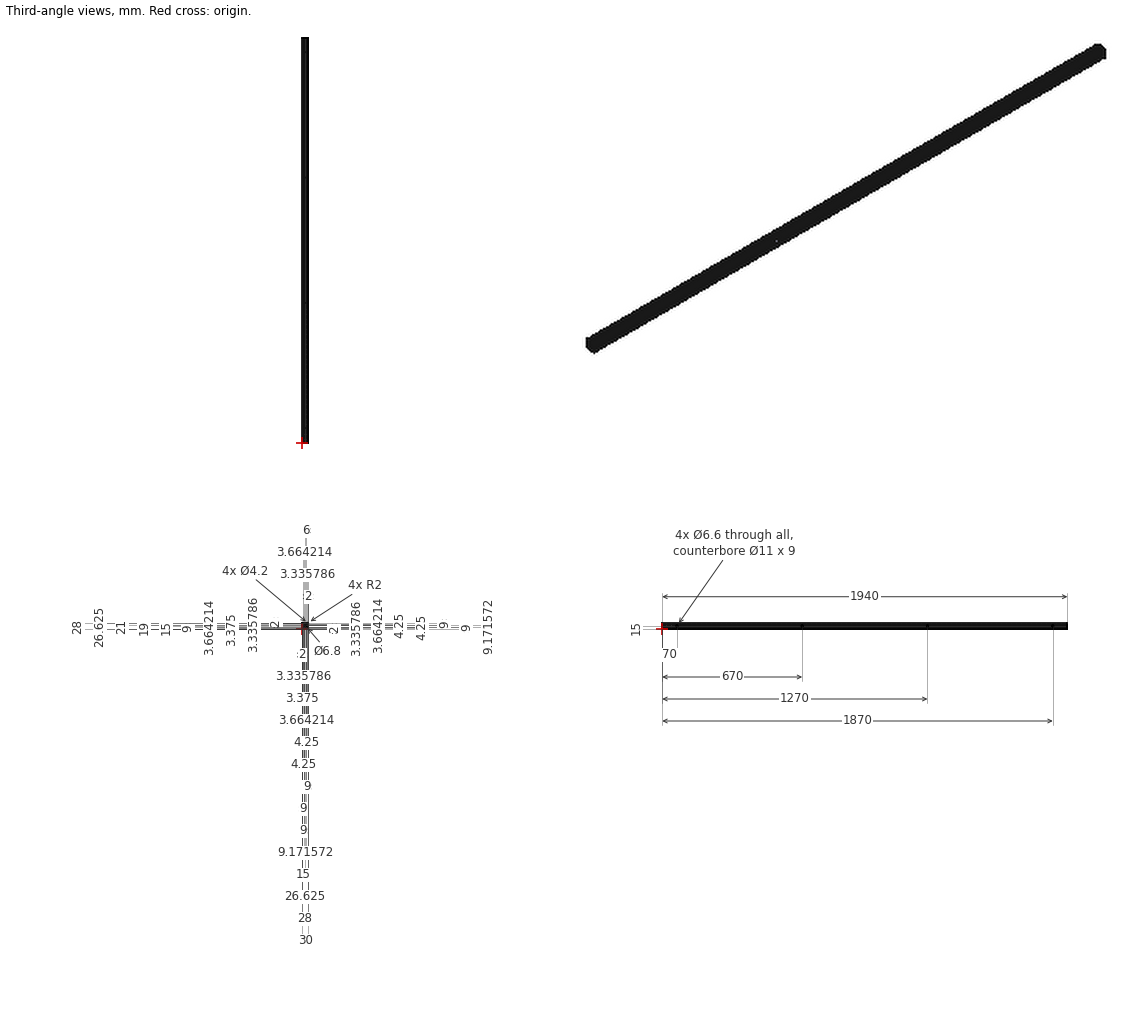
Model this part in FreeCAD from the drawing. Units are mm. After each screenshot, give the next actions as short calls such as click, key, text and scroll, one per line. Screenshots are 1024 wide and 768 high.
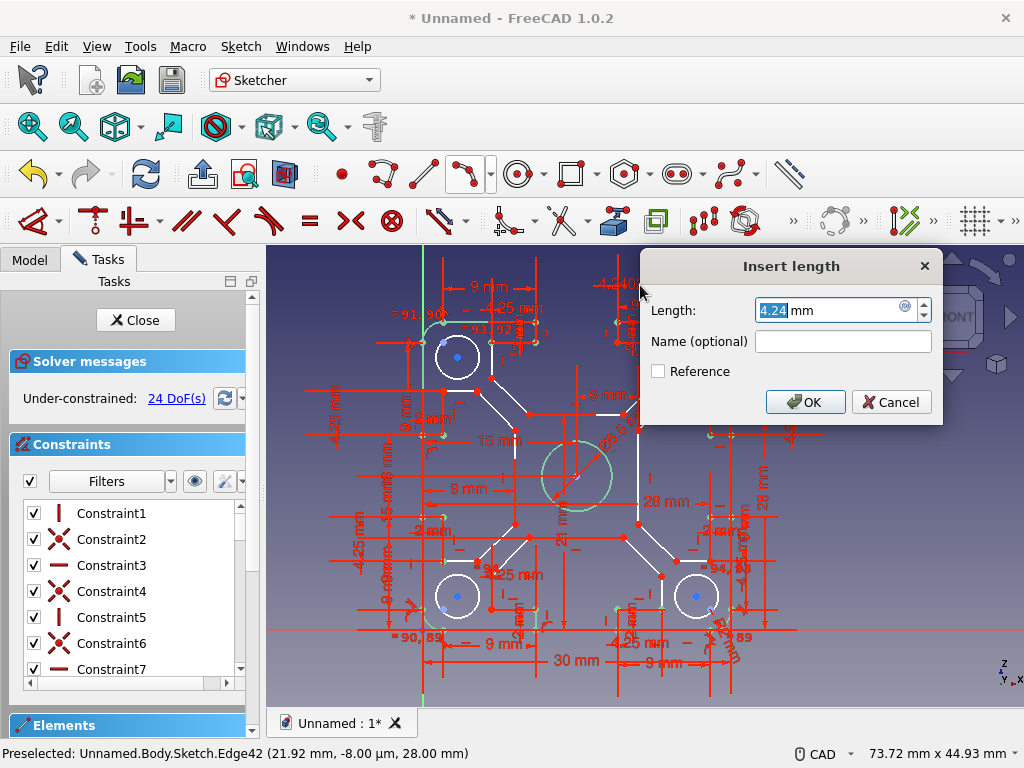
text(4.25)
key(Return)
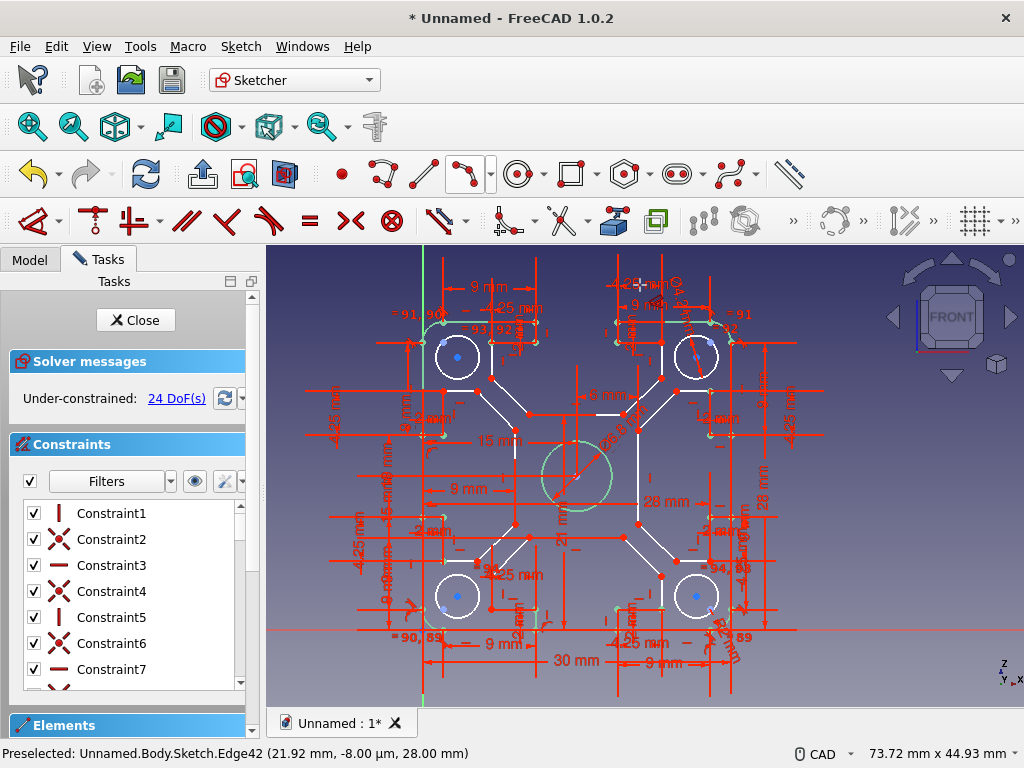
click(458, 357)
click(440, 664)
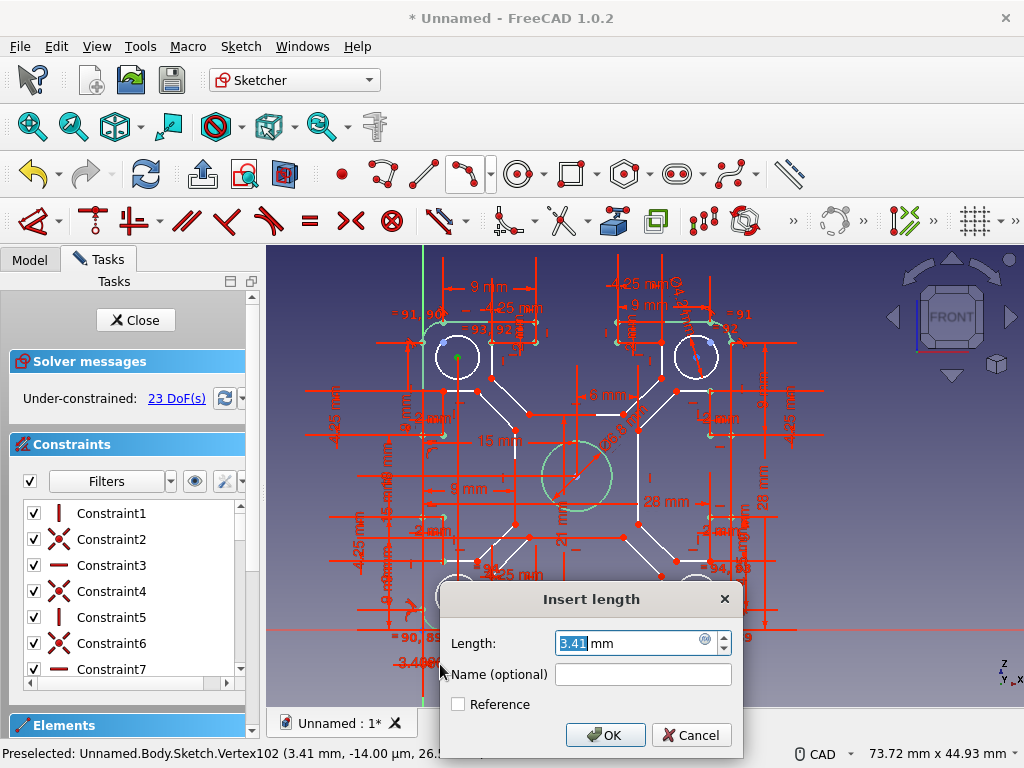
text(3.375)
key(Return)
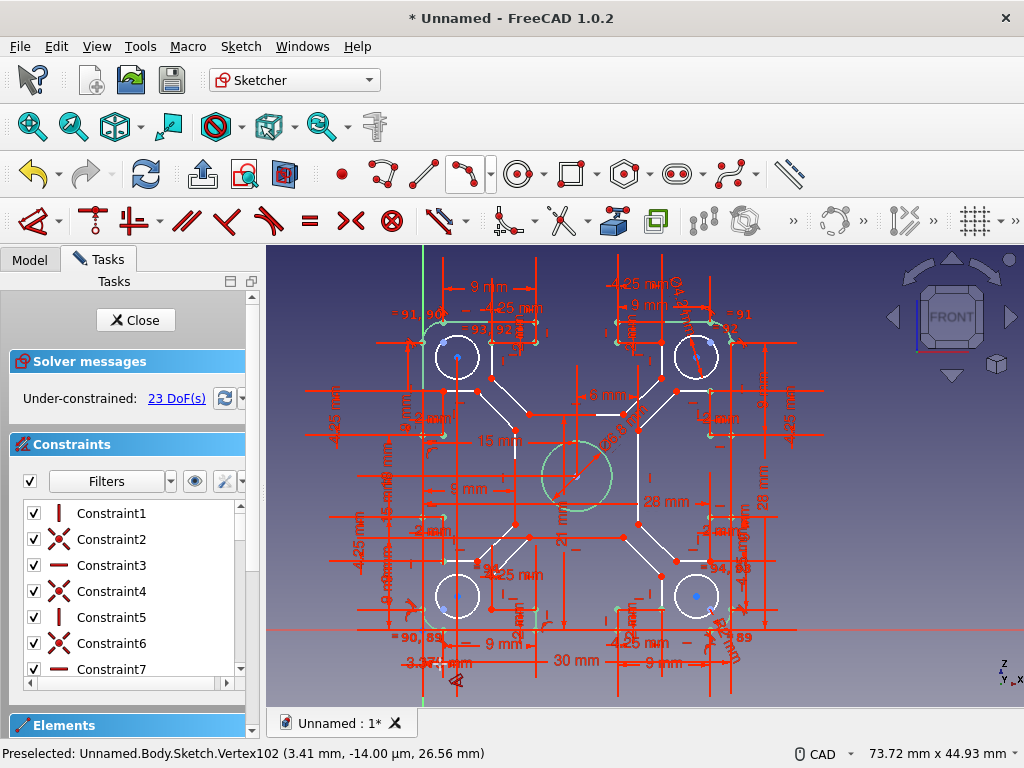
click(697, 596)
click(389, 613)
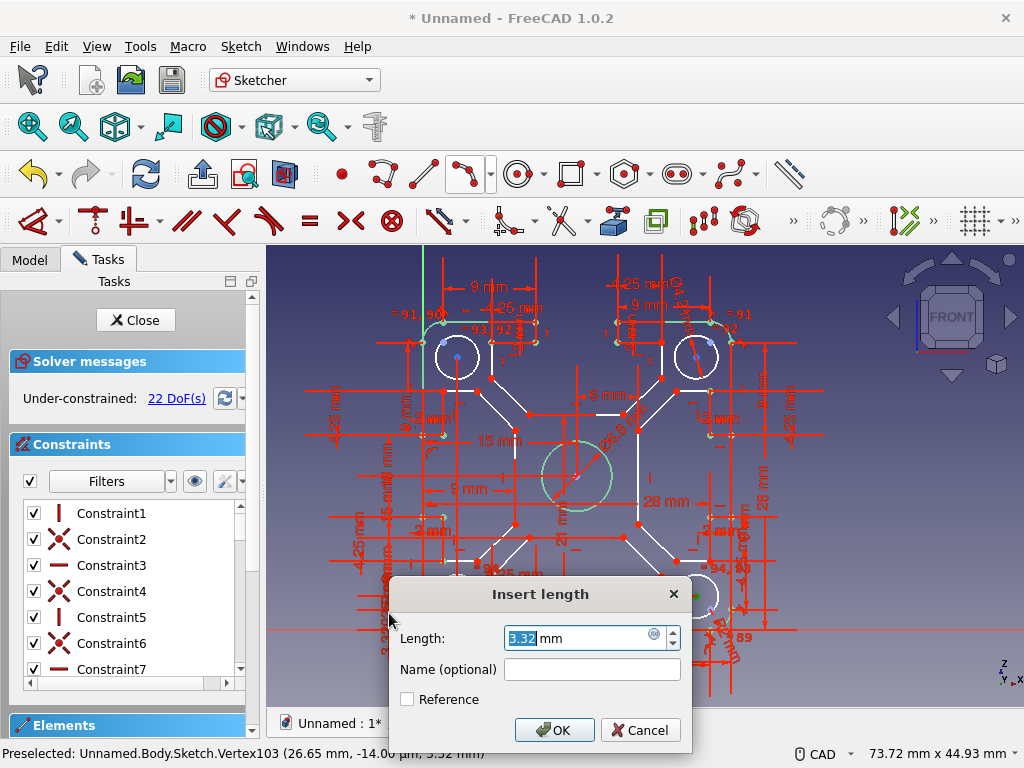
text(3.375)
key(Return)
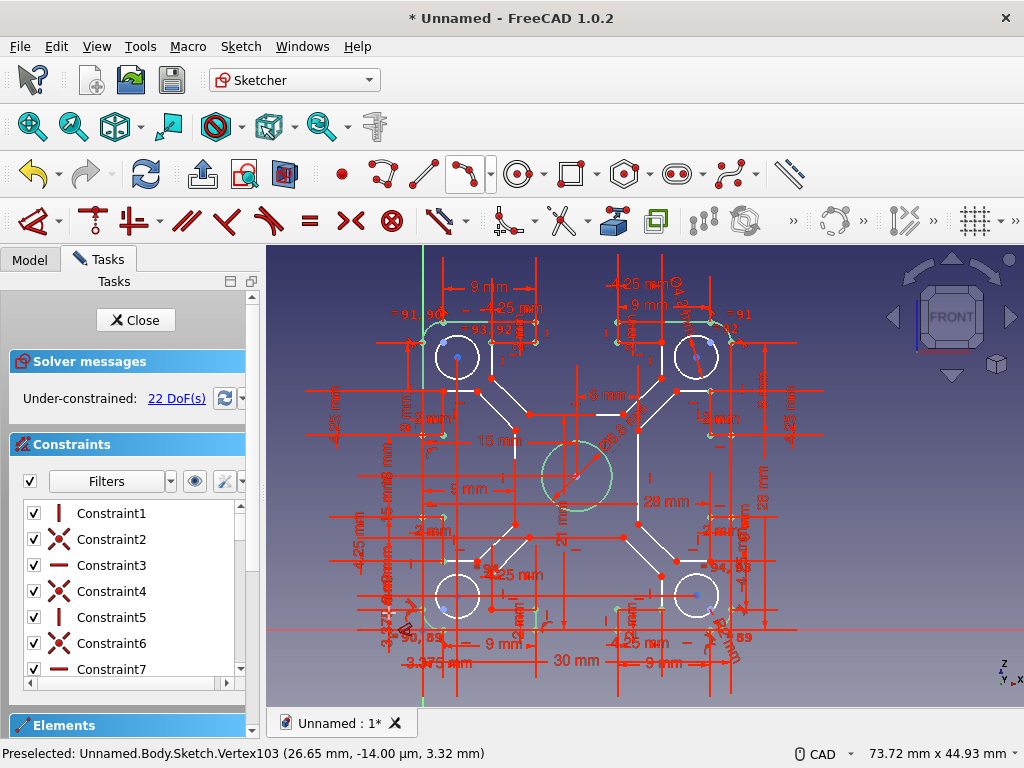
click(458, 596)
click(432, 562)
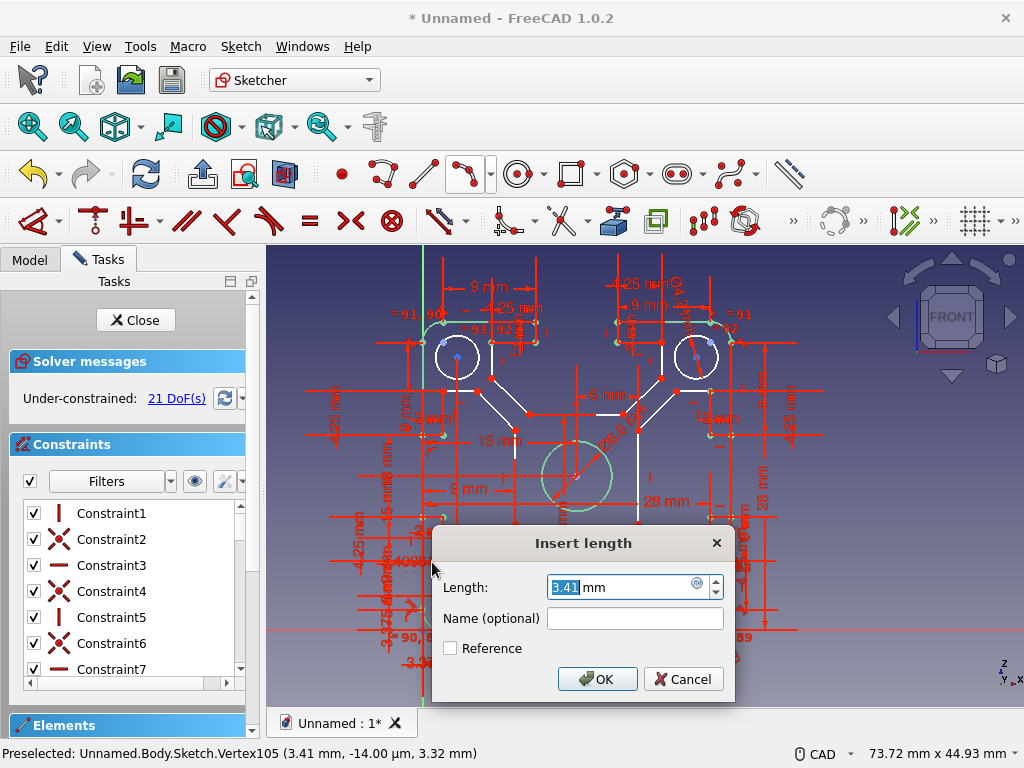
text(3.375)
key(Return)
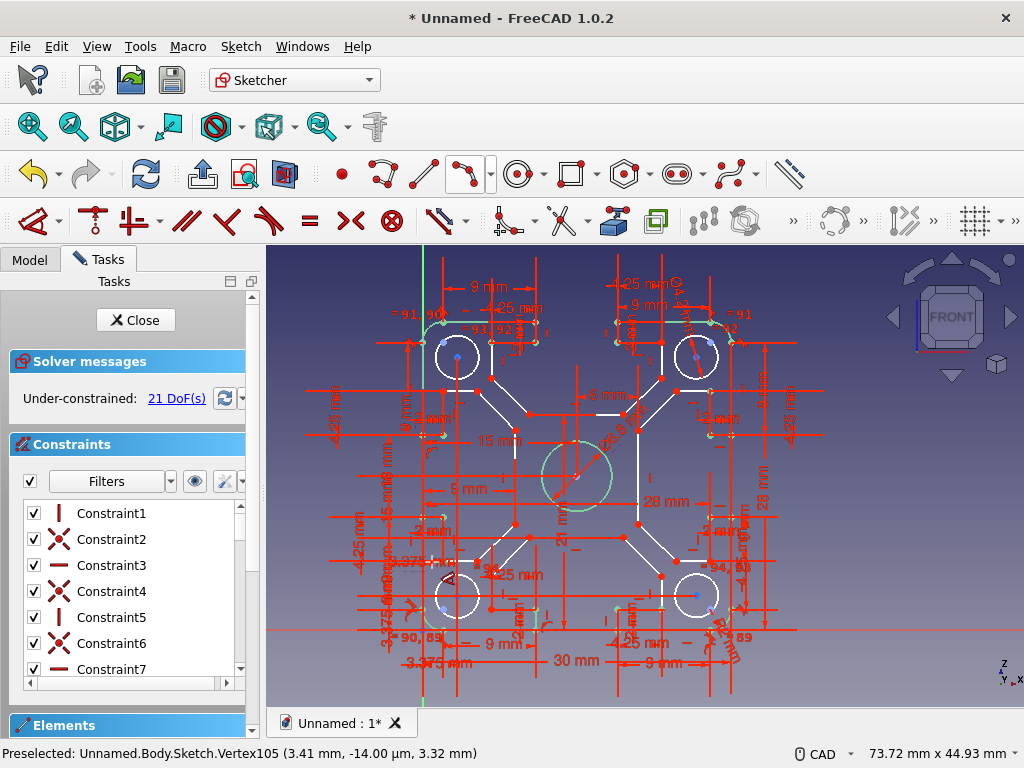
click(457, 596)
click(317, 613)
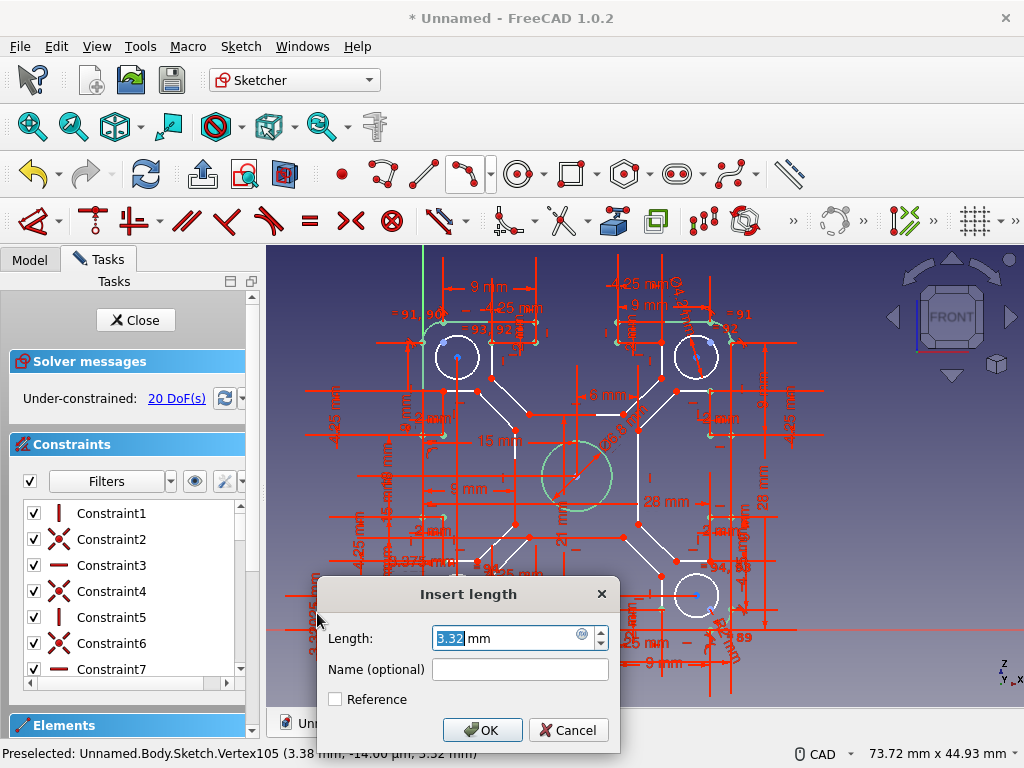
text(3.375)
key(Return)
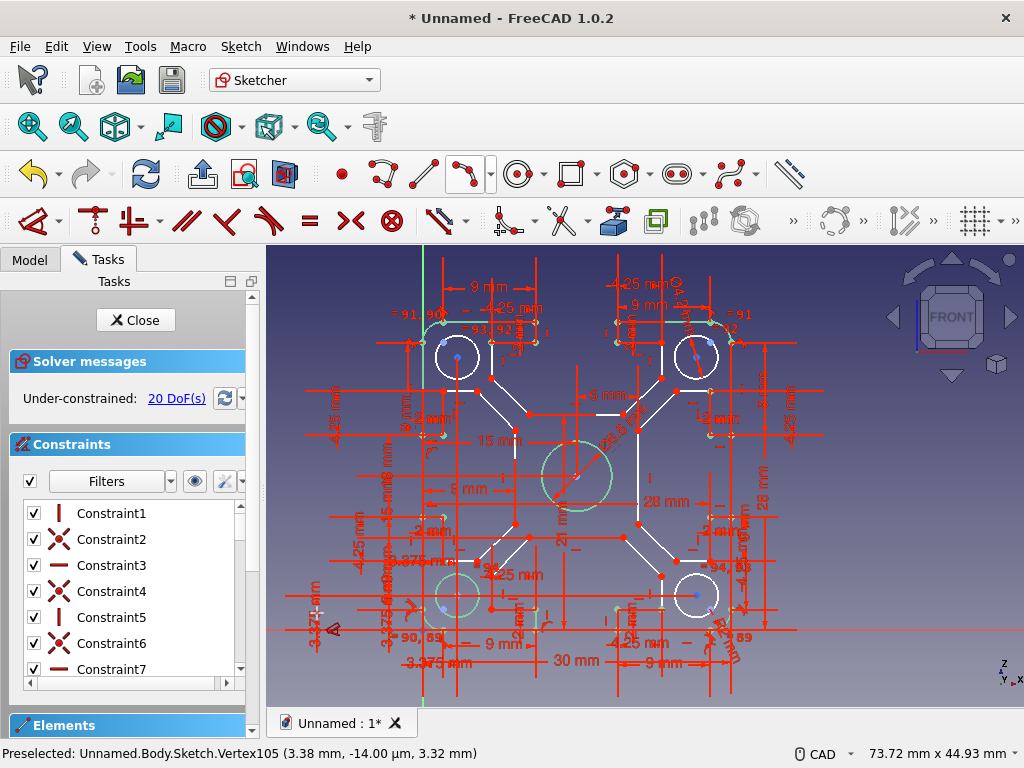
click(696, 357)
click(559, 275)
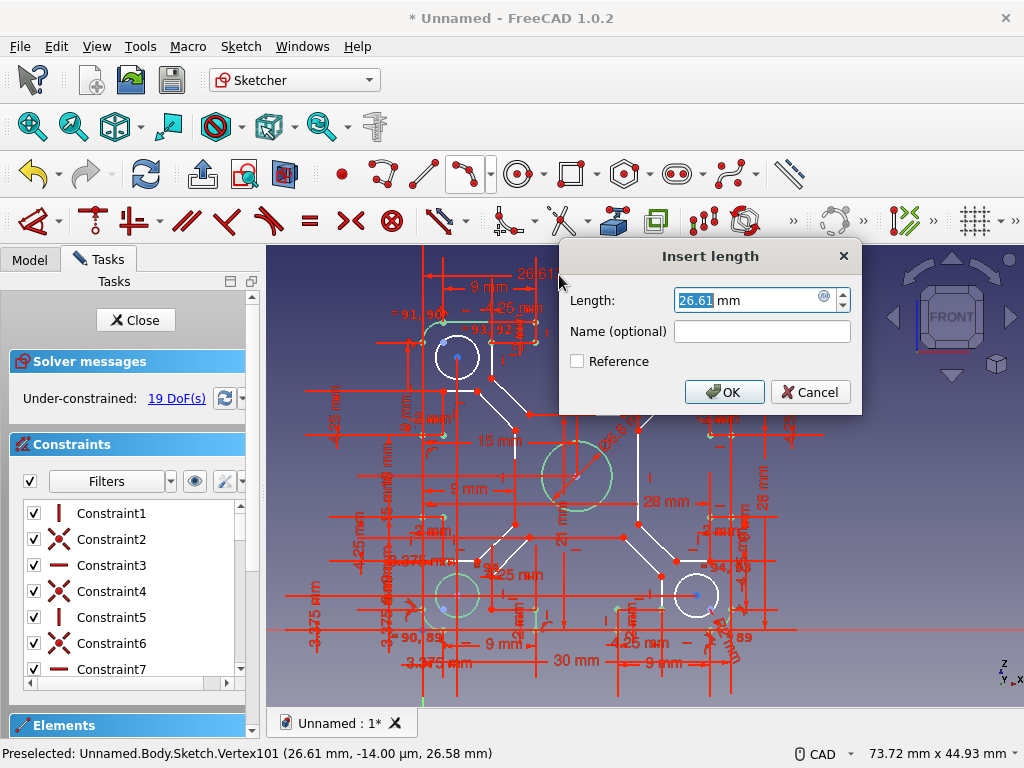
text(26.625)
key(Return)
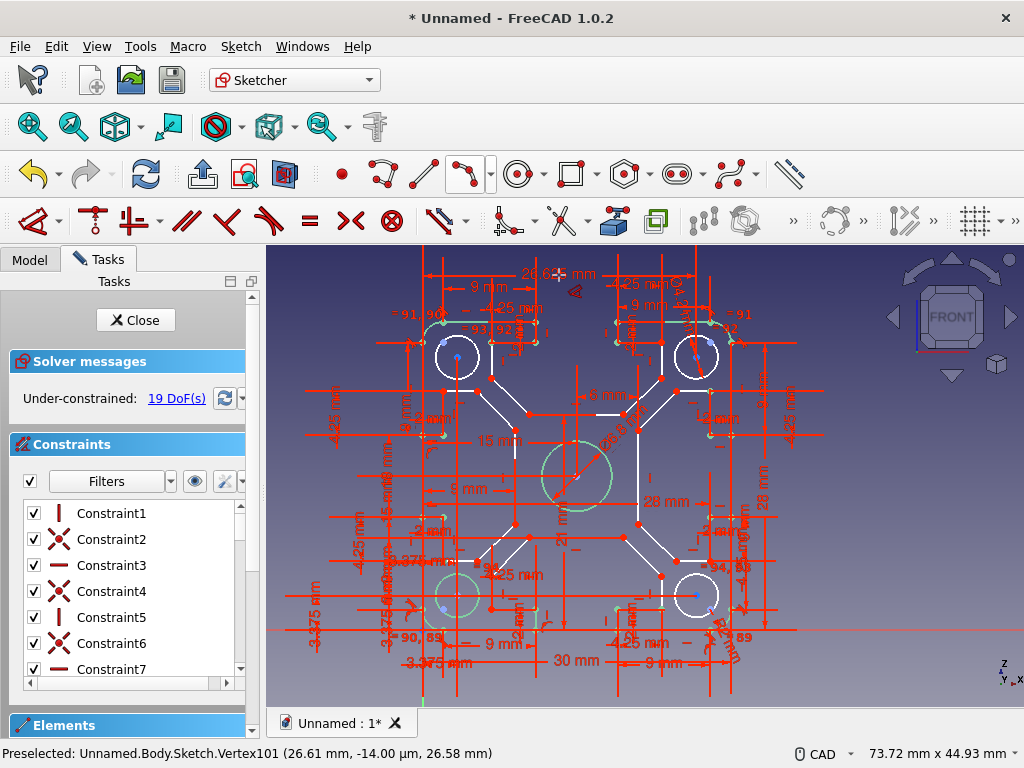
click(696, 357)
click(754, 589)